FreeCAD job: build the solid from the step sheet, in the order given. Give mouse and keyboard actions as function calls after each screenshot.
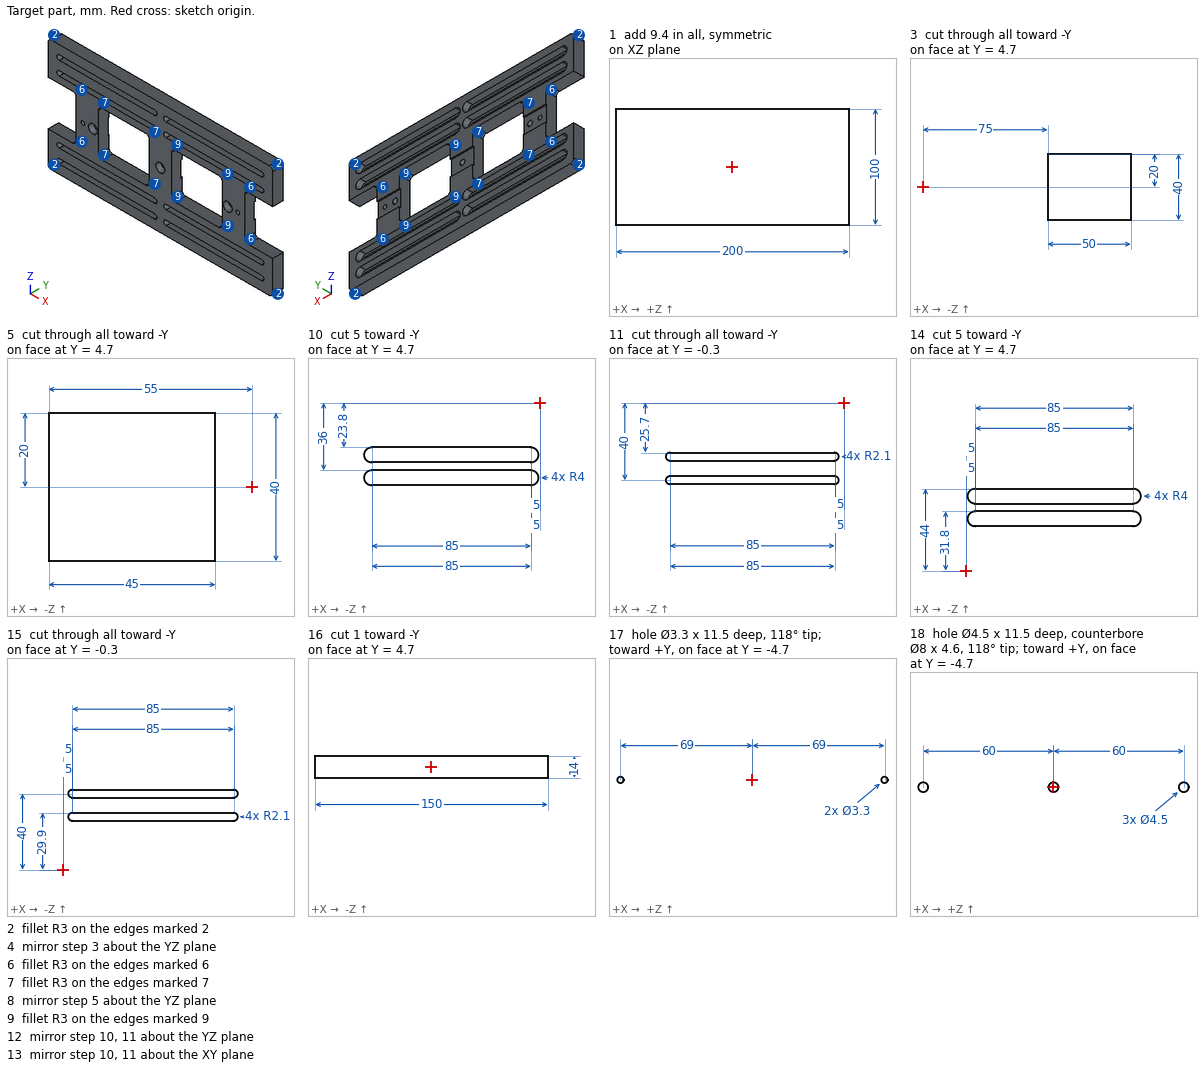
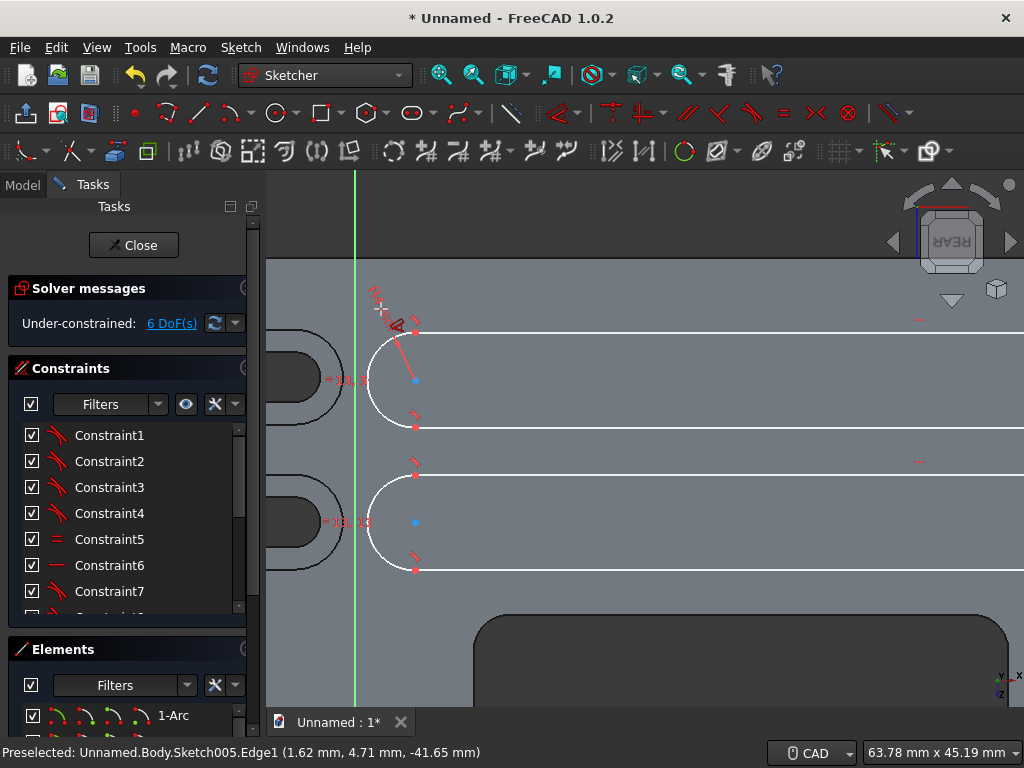
click(717, 333)
click(637, 299)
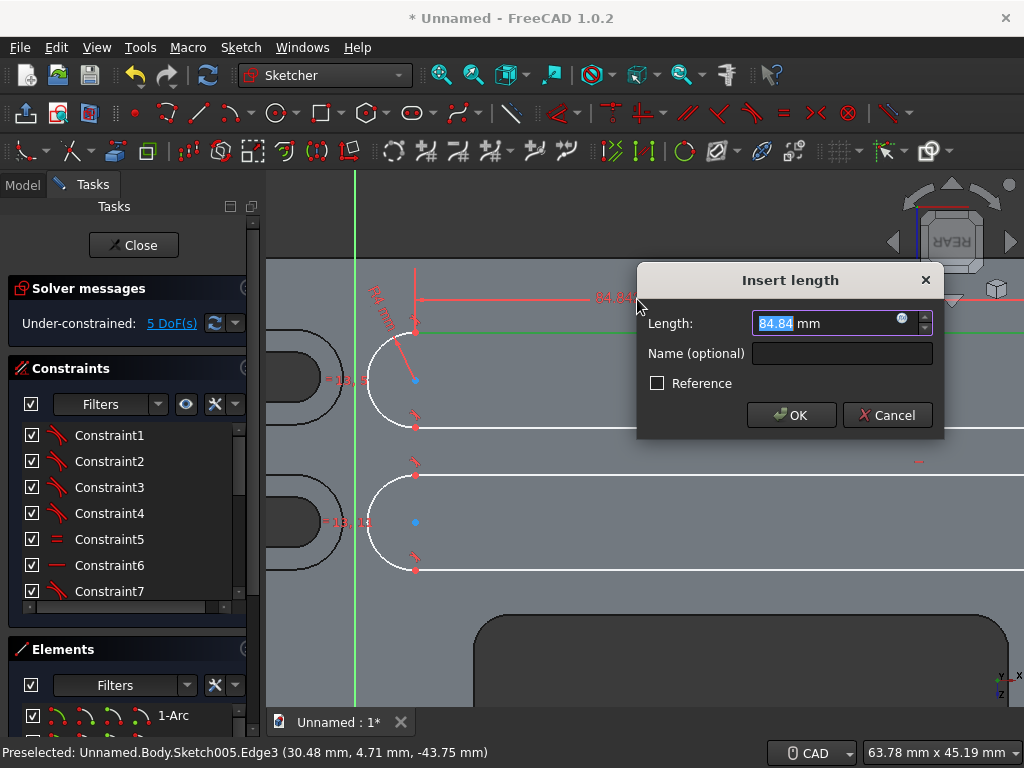
text(85)
key(Return)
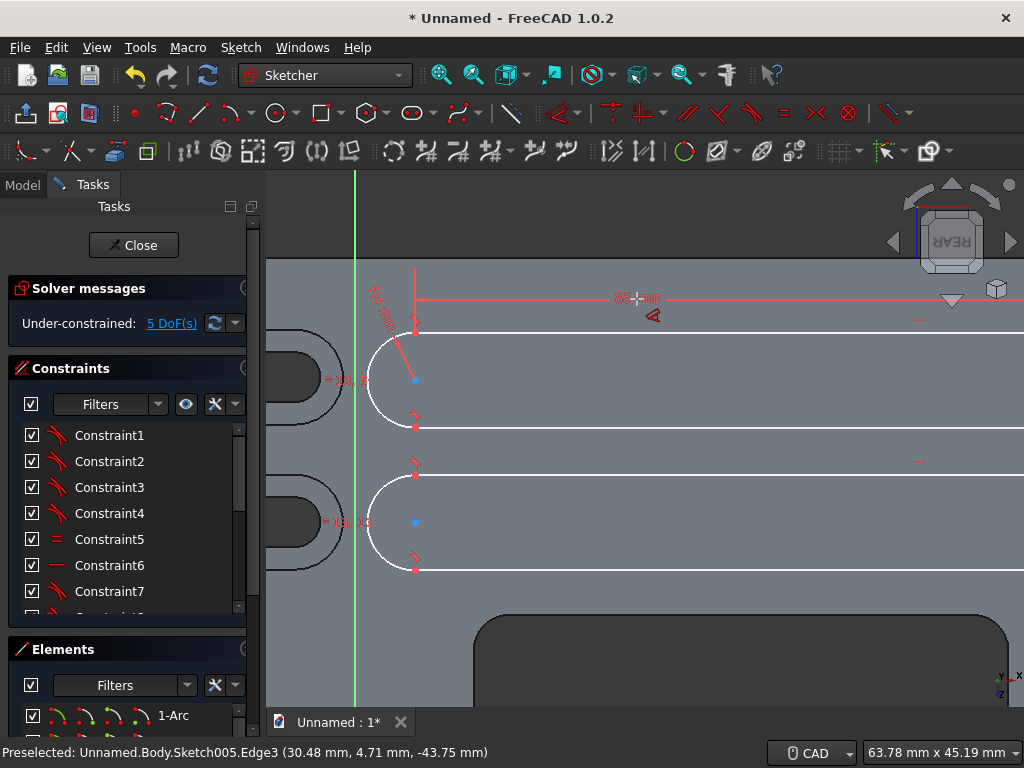
click(718, 475)
click(637, 441)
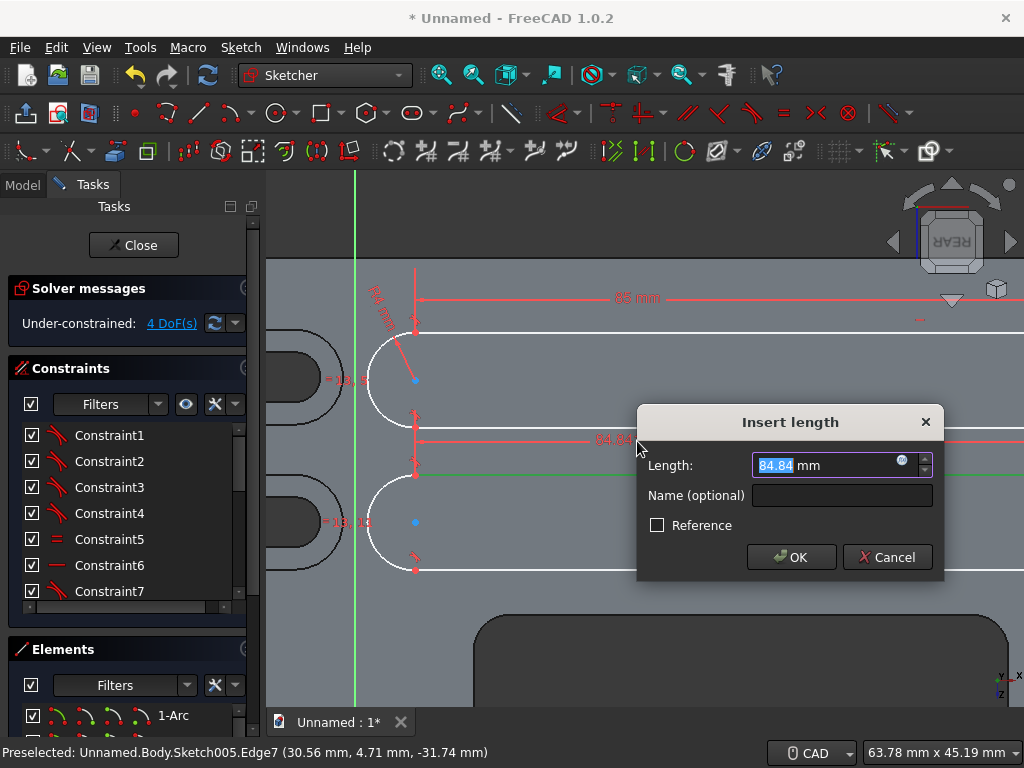
text(85)
key(Return)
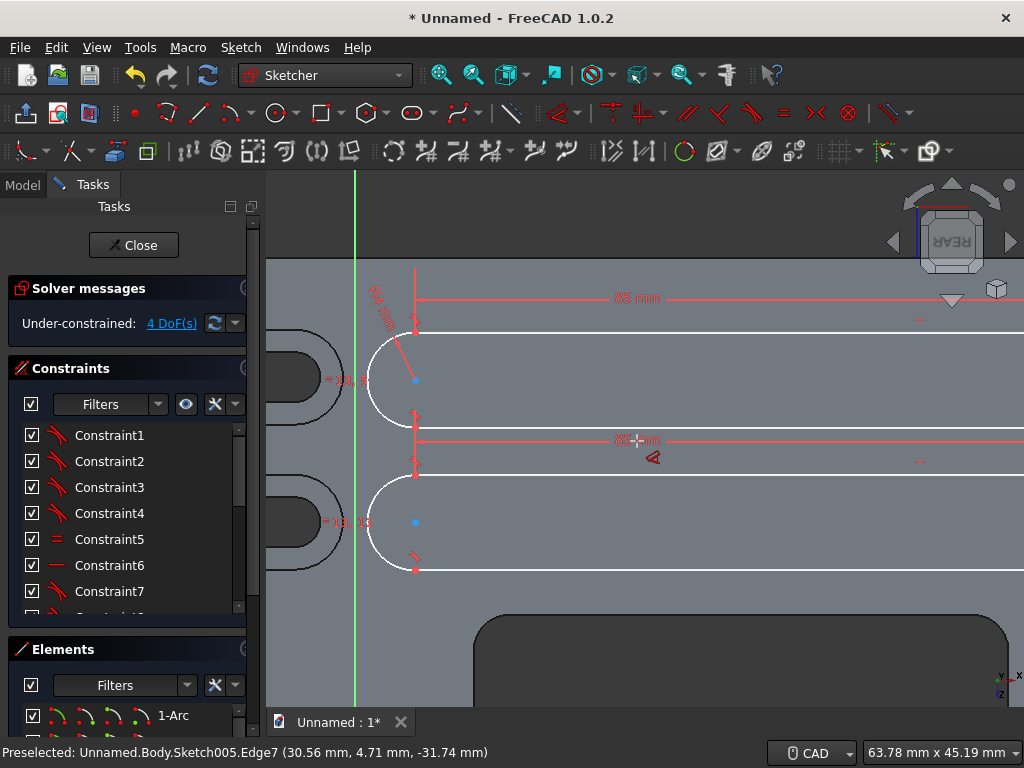
click(415, 333)
click(385, 275)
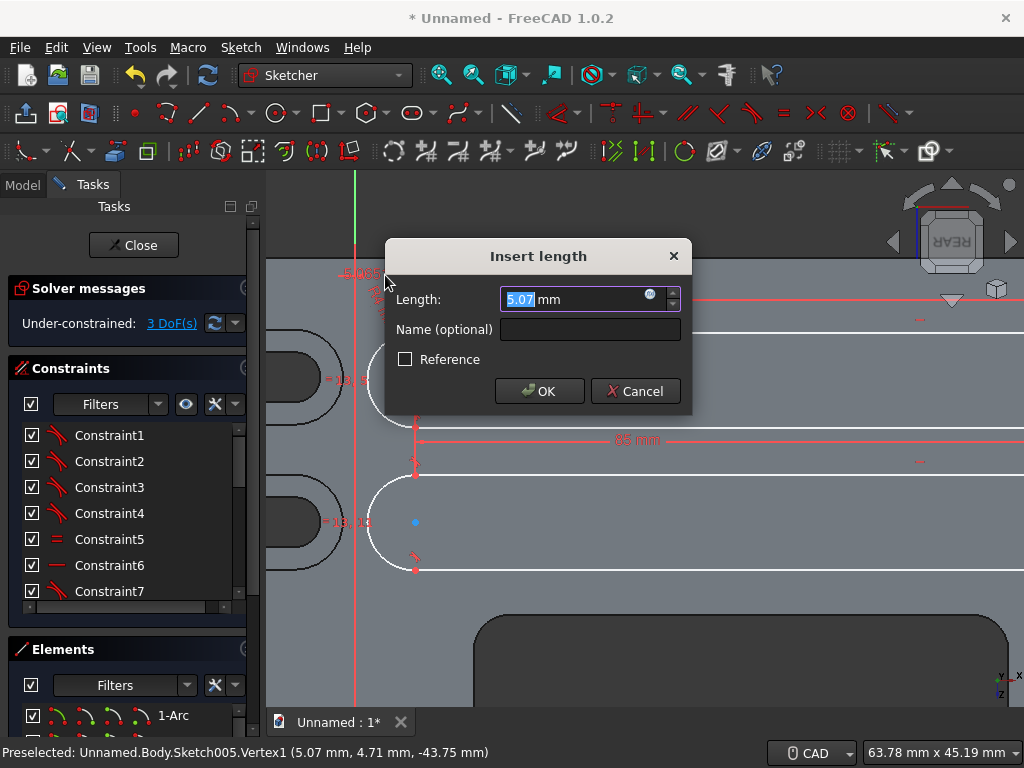
text(5)
key(Return)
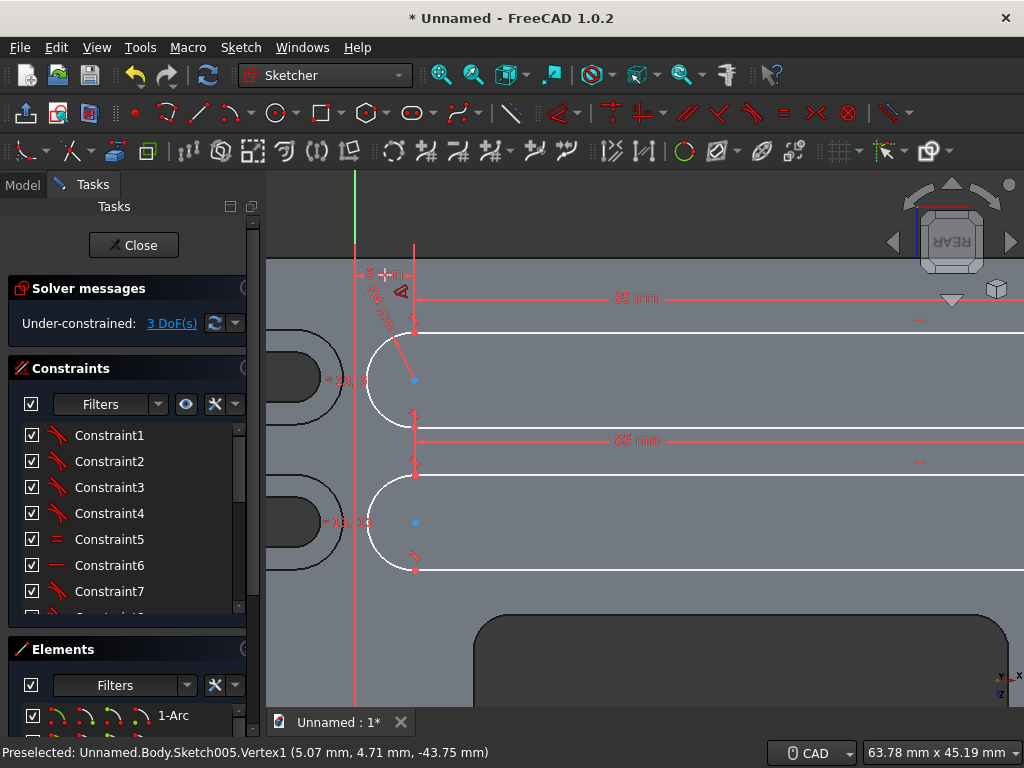
click(415, 475)
click(385, 441)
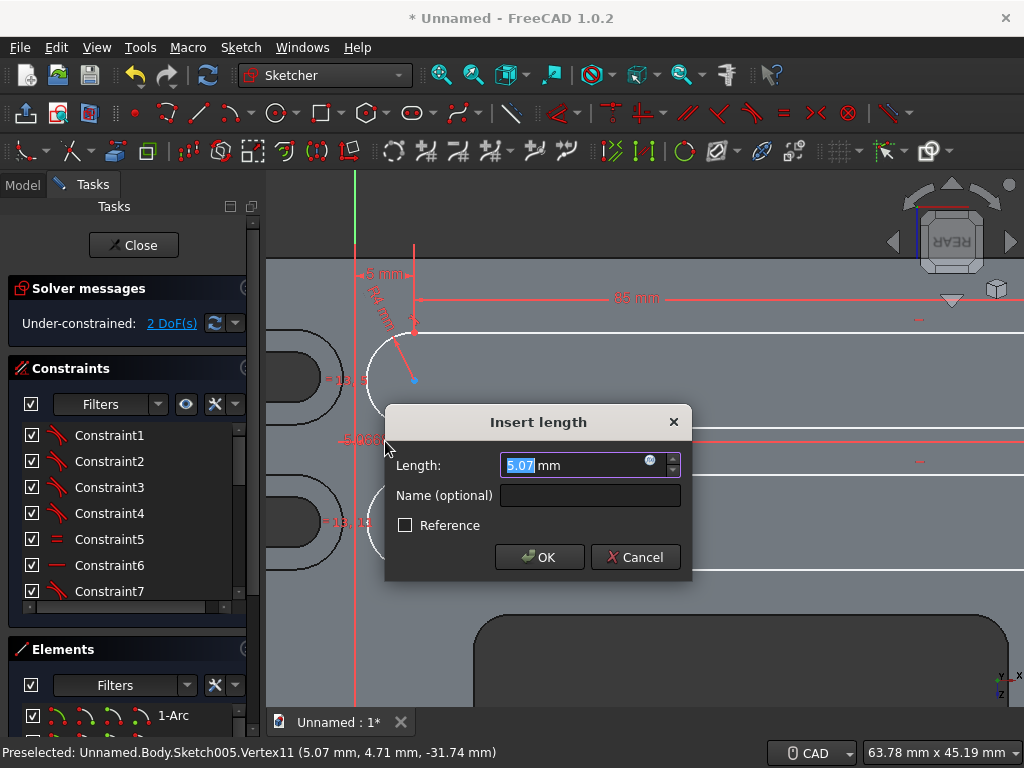
text(5)
key(Return)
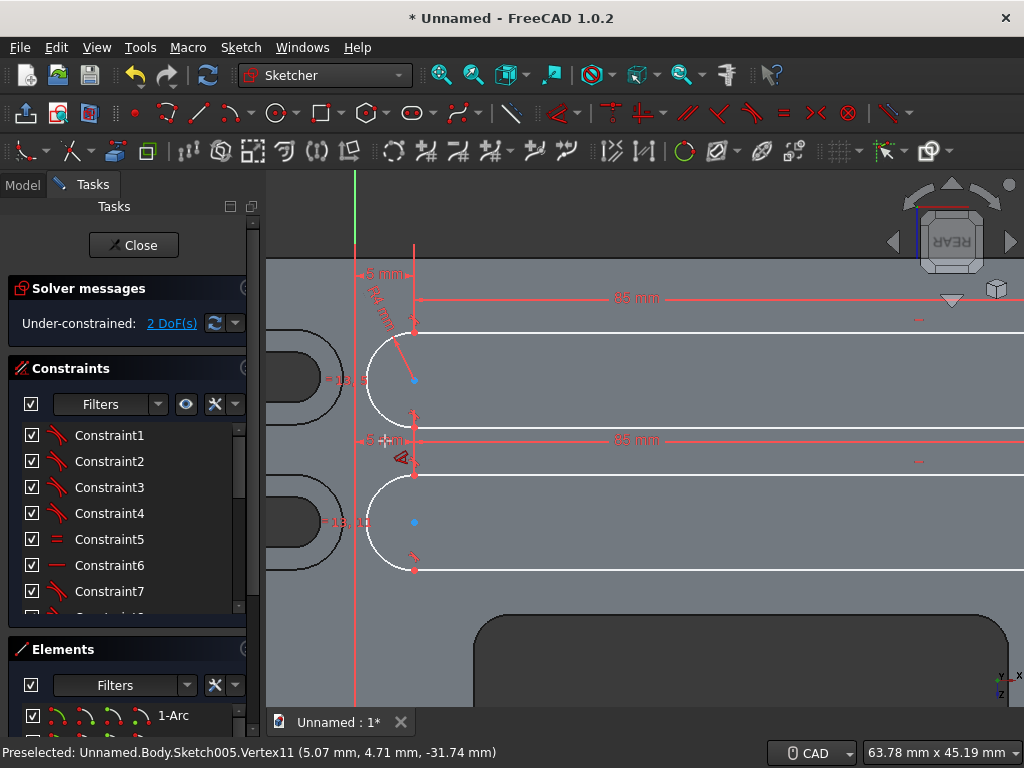
click(414, 333)
click(321, 506)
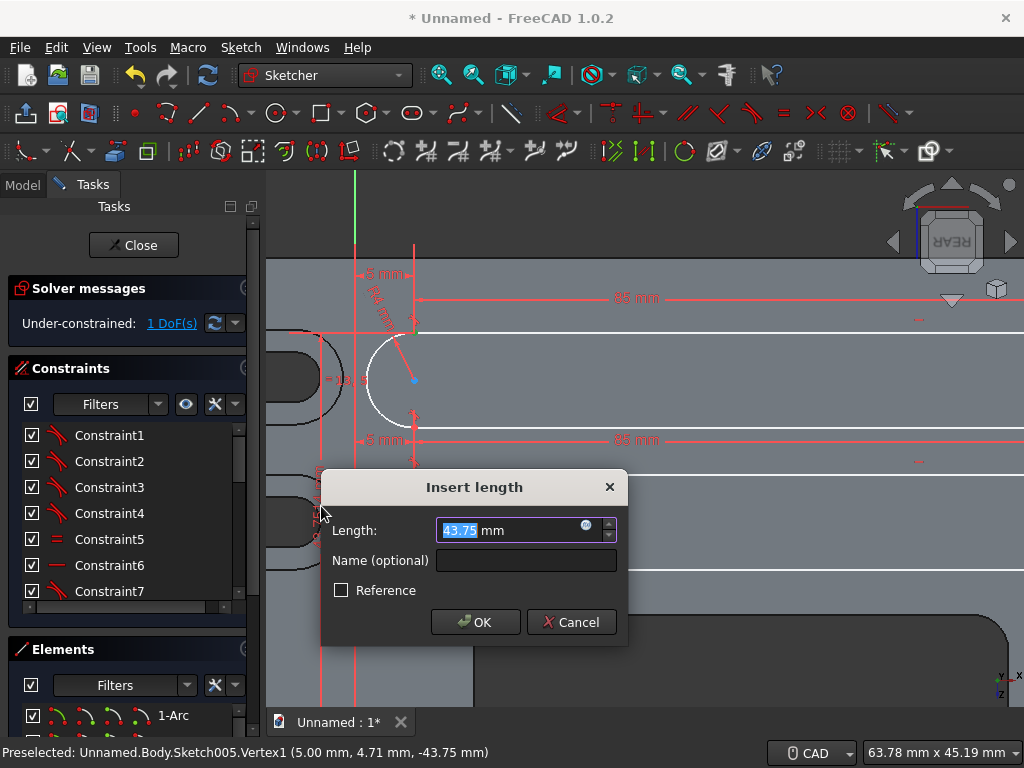
text(44)
key(Return)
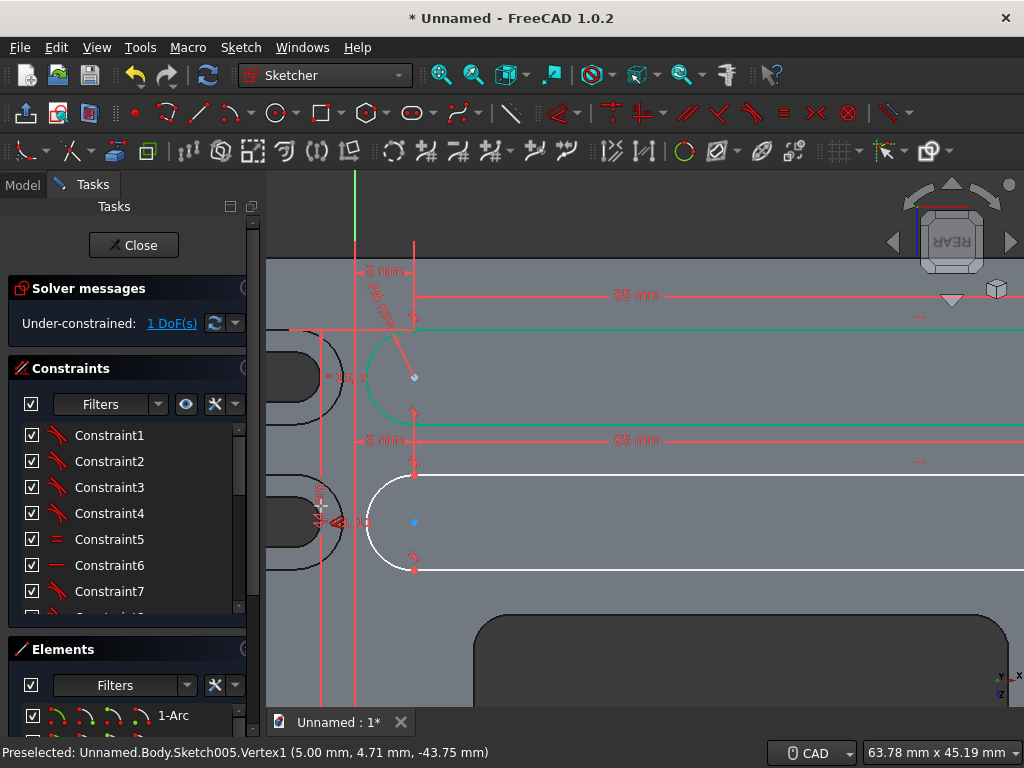
click(414, 475)
click(321, 577)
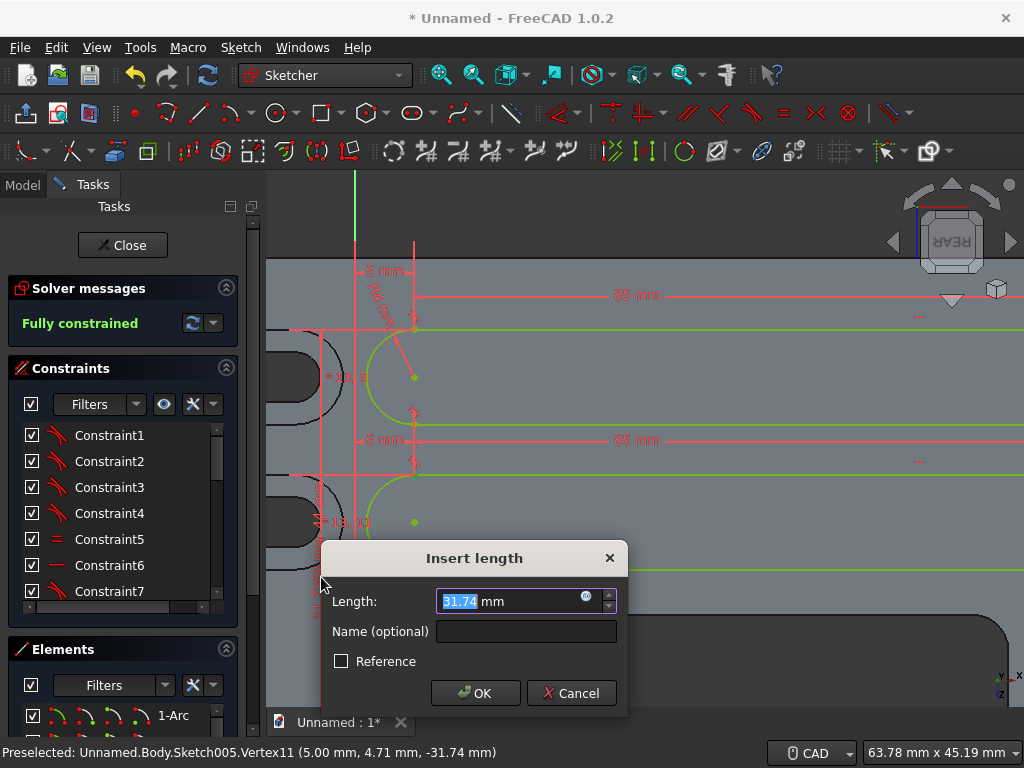
text(31.8)
key(Return)
key(Escape)